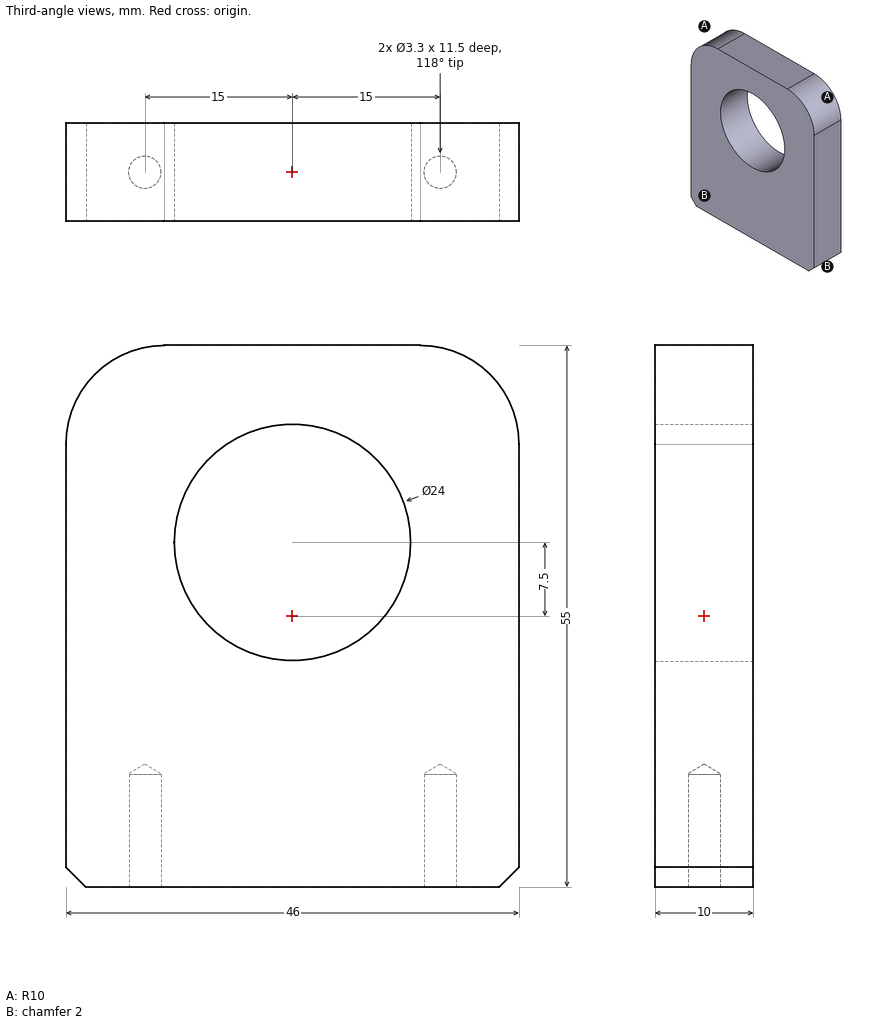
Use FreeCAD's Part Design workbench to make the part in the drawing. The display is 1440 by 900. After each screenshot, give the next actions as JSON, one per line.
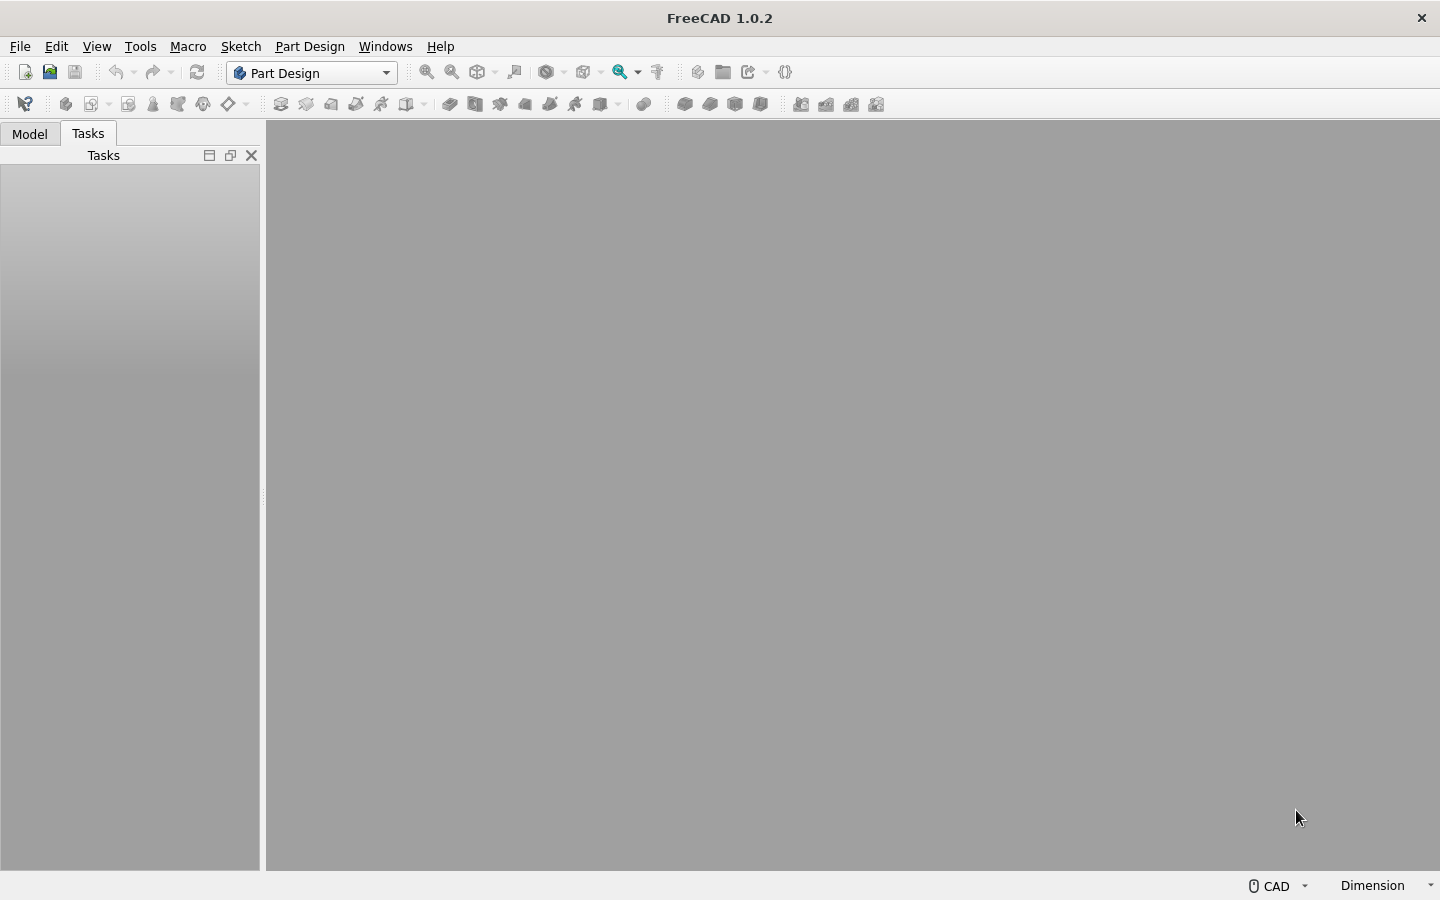
{"action": "left_click", "coordinate": [25, 72]}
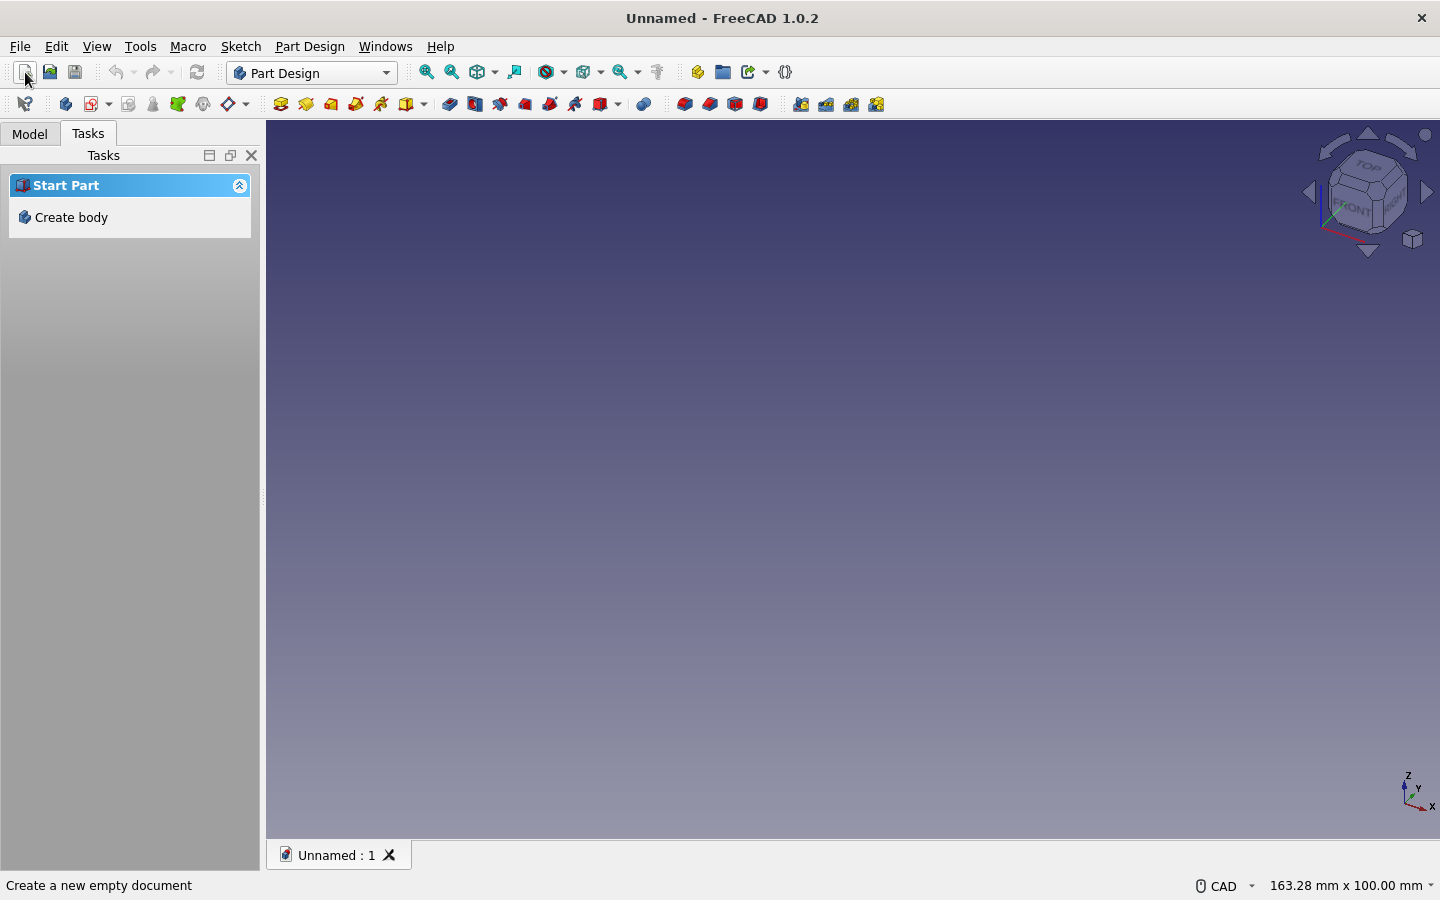
{"action": "left_click", "coordinate": [90, 104]}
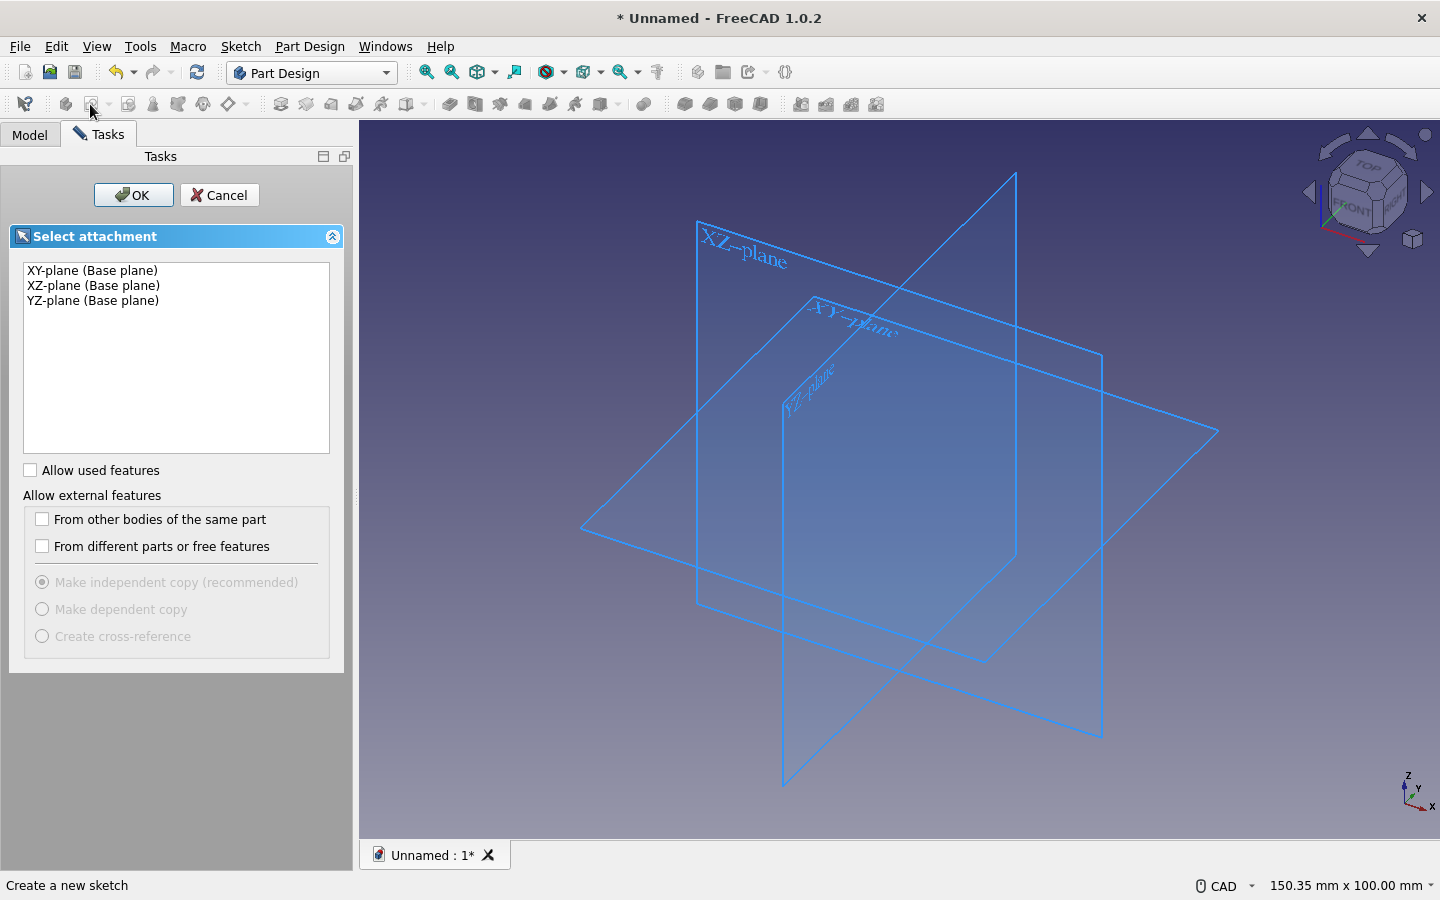
{"action": "left_click", "coordinate": [84, 286]}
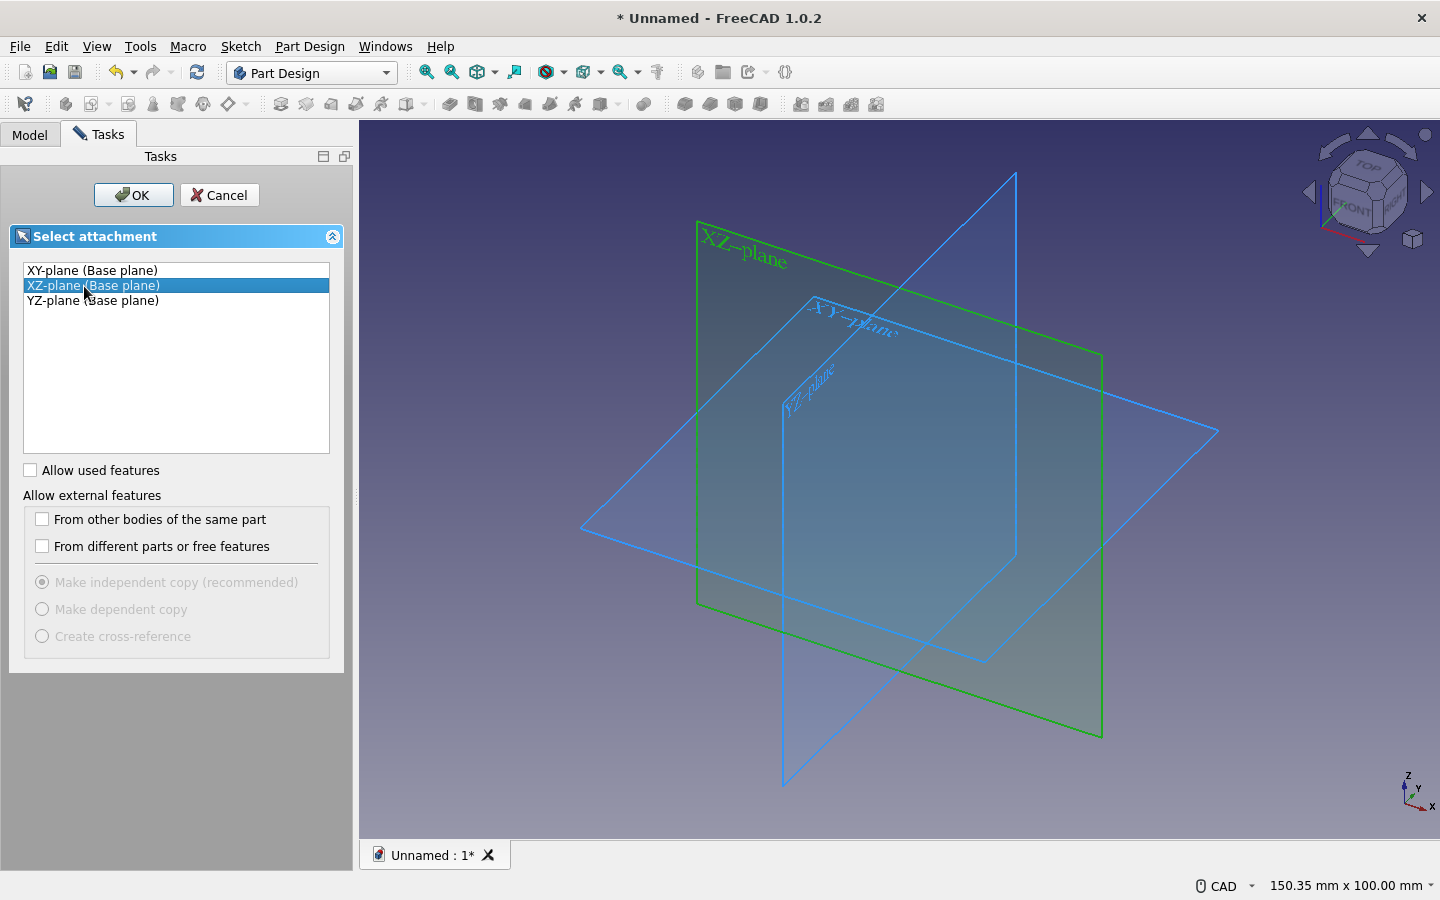
{"action": "left_click", "coordinate": [134, 195]}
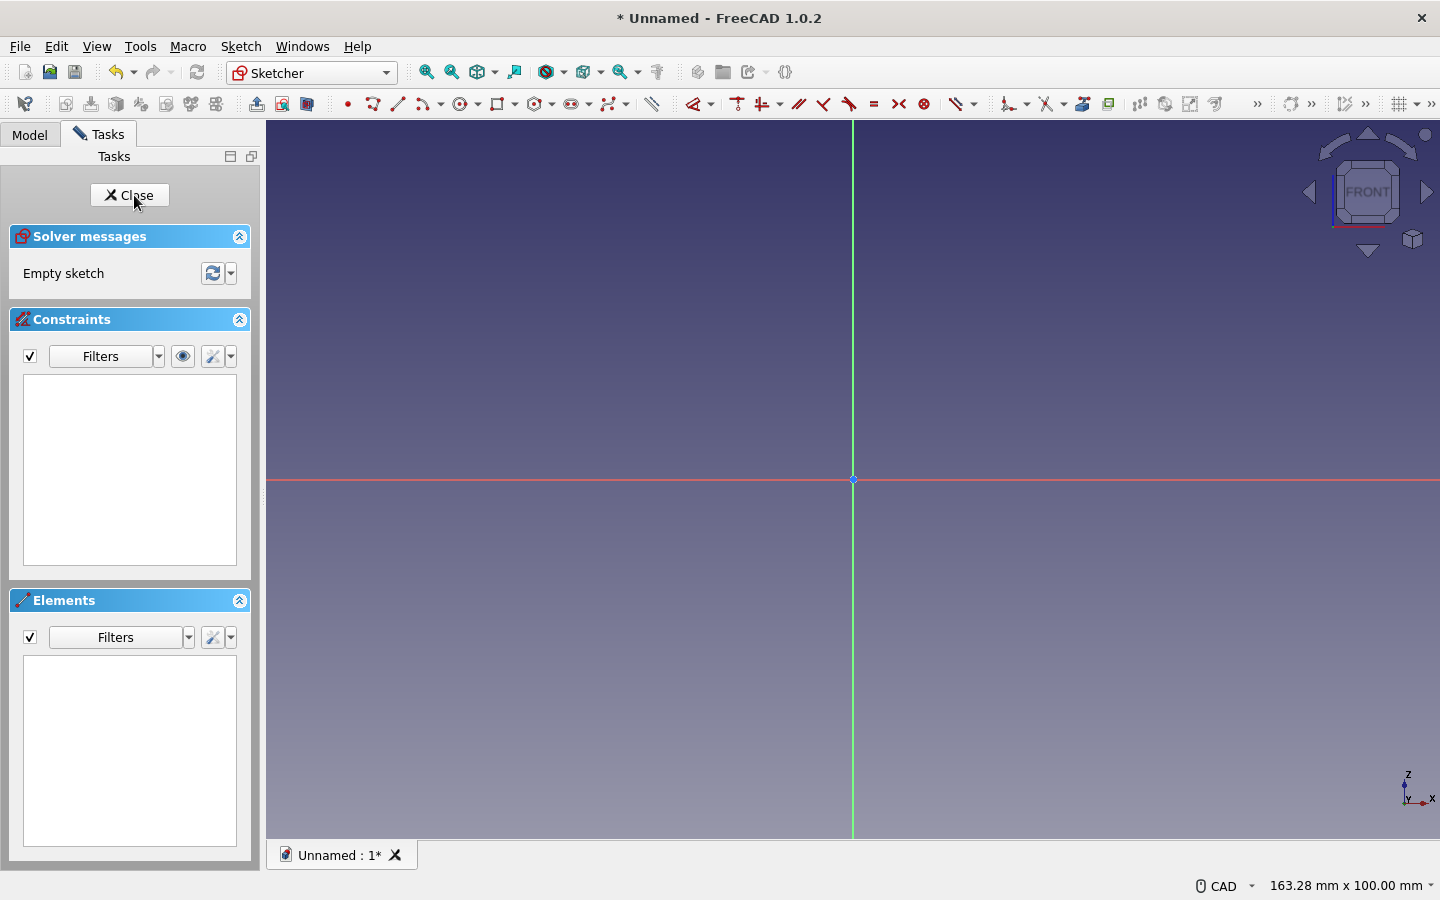
{"action": "key", "text": "g v"}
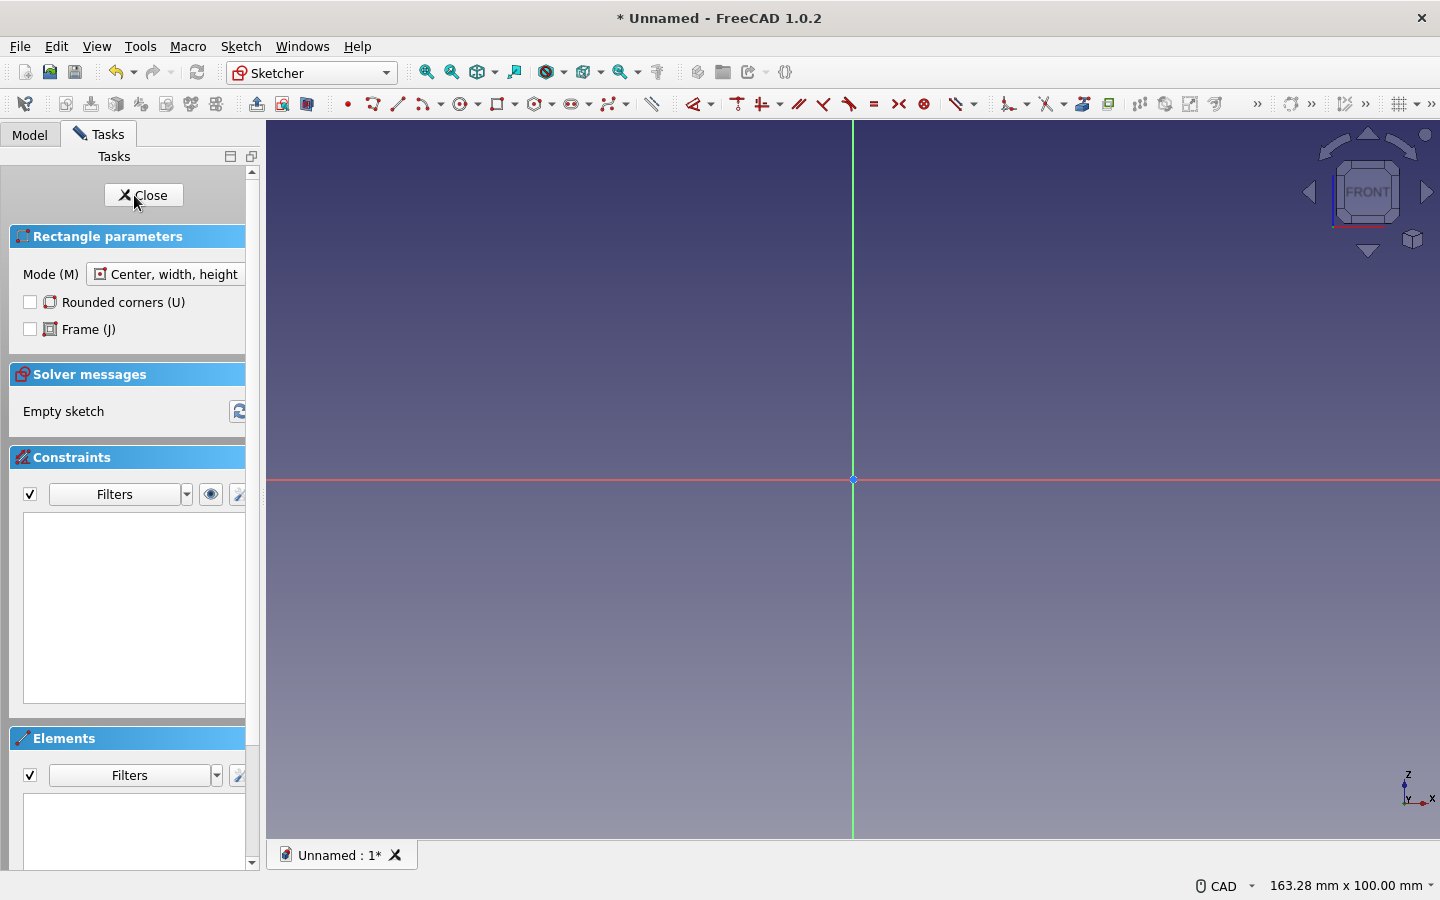
{"action": "left_click", "coordinate": [853, 480]}
{"action": "left_click", "coordinate": [1018, 282]}
{"action": "key", "text": "Escape"}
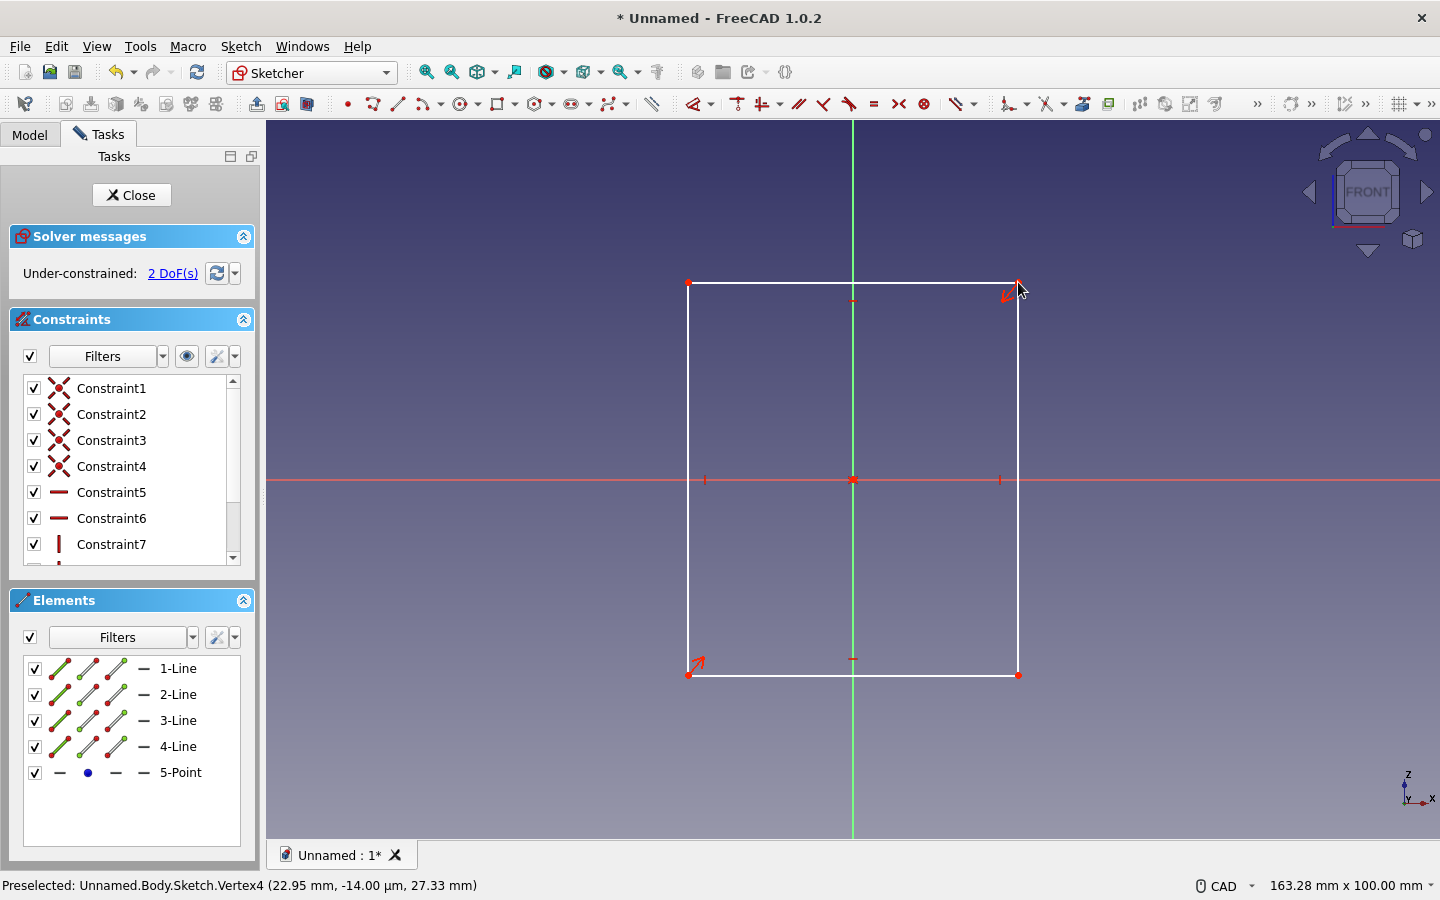
{"action": "left_click", "coordinate": [692, 104]}